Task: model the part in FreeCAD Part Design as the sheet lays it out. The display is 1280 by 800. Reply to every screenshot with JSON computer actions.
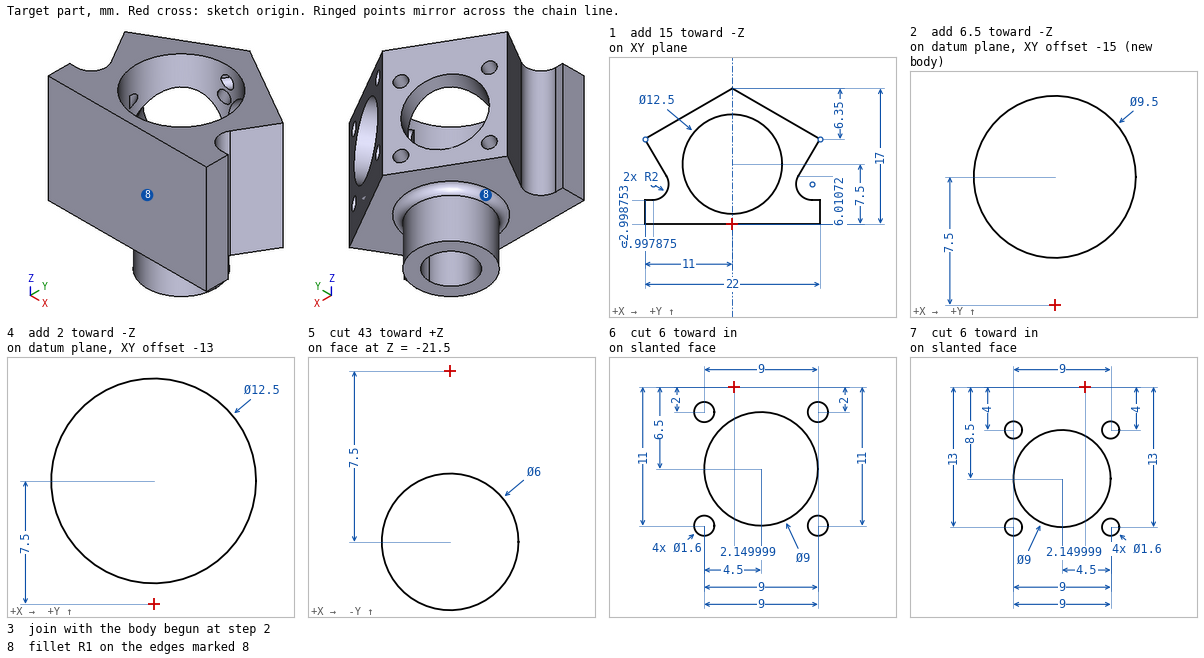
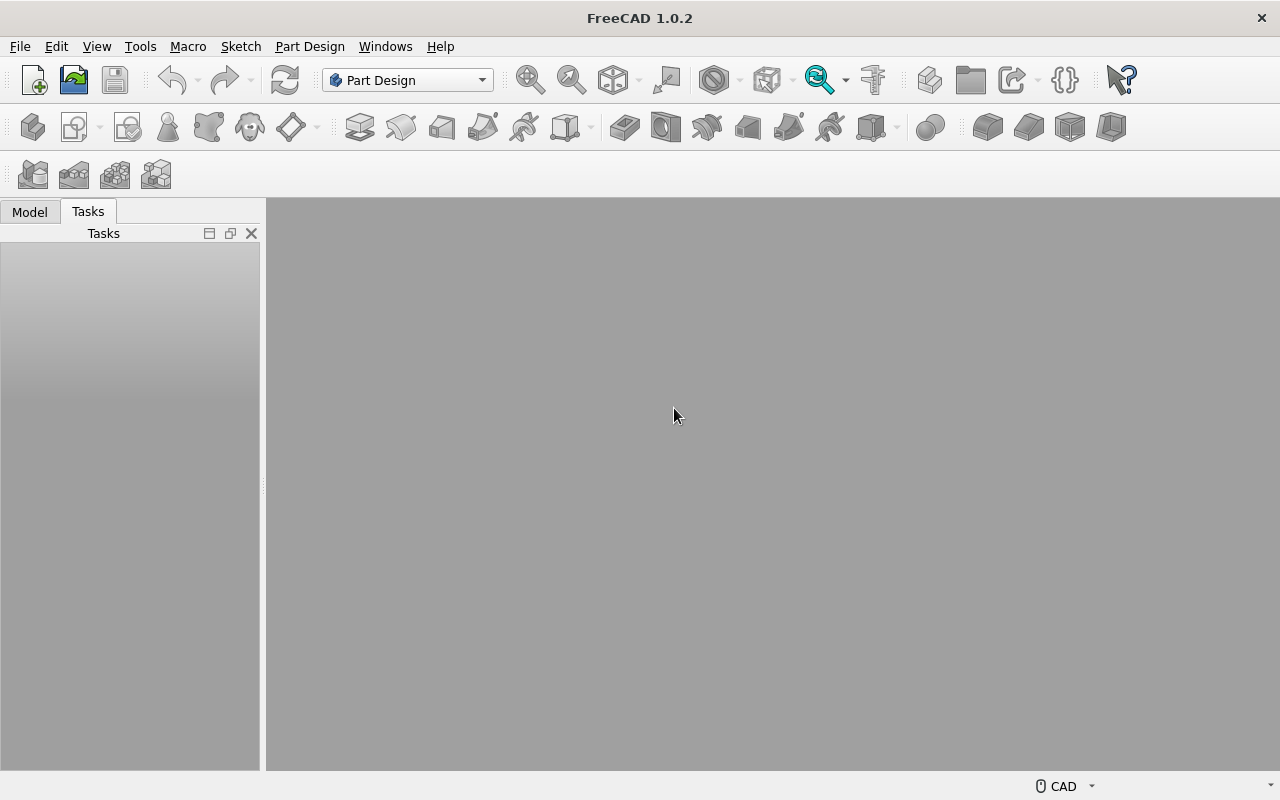
{"action": "left_click", "coordinate": [33, 80]}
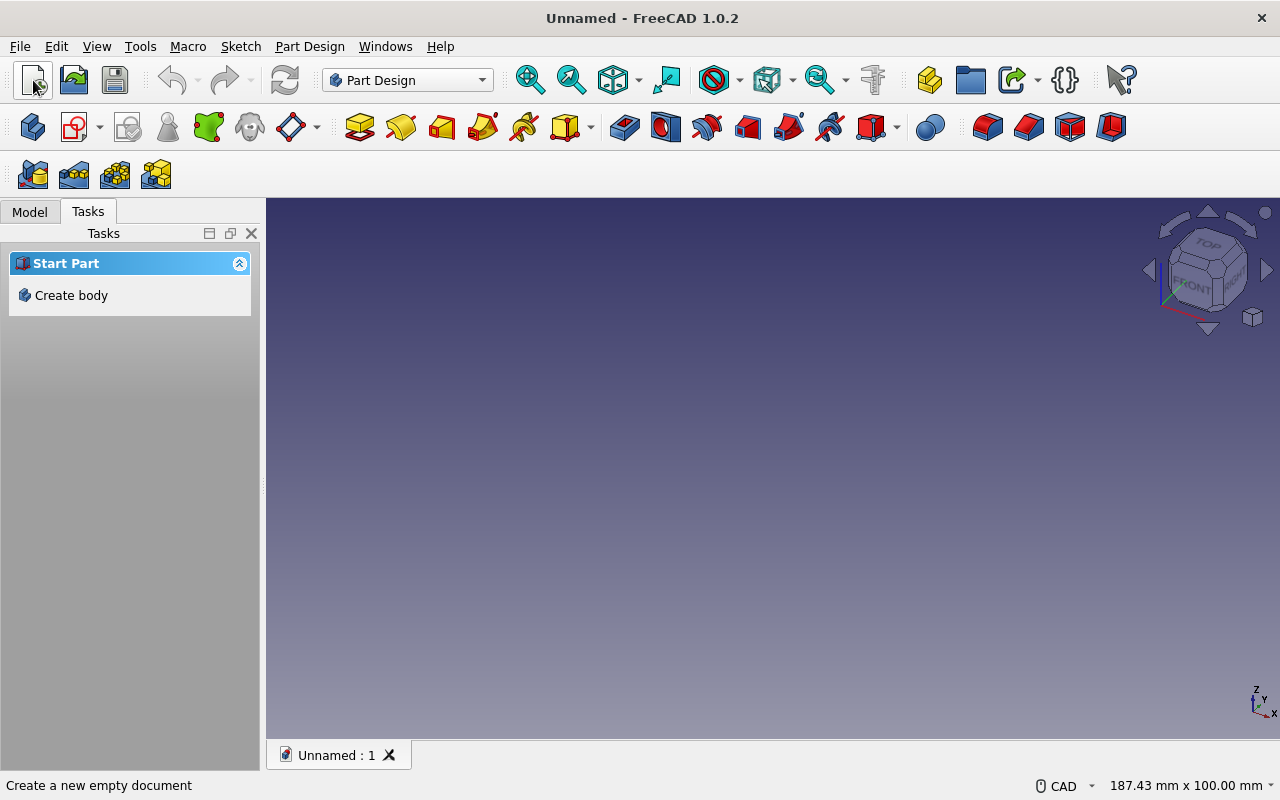
{"action": "left_click", "coordinate": [74, 128]}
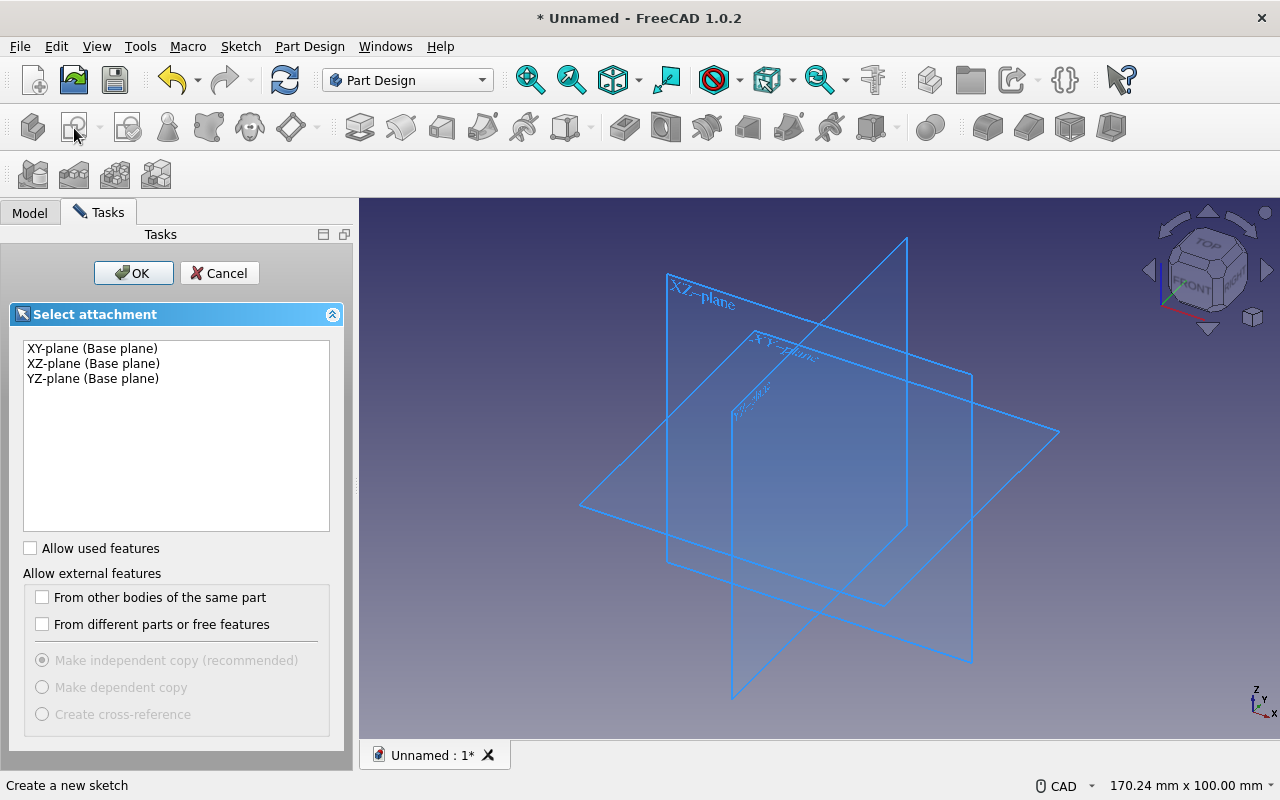
{"action": "left_click", "coordinate": [84, 348]}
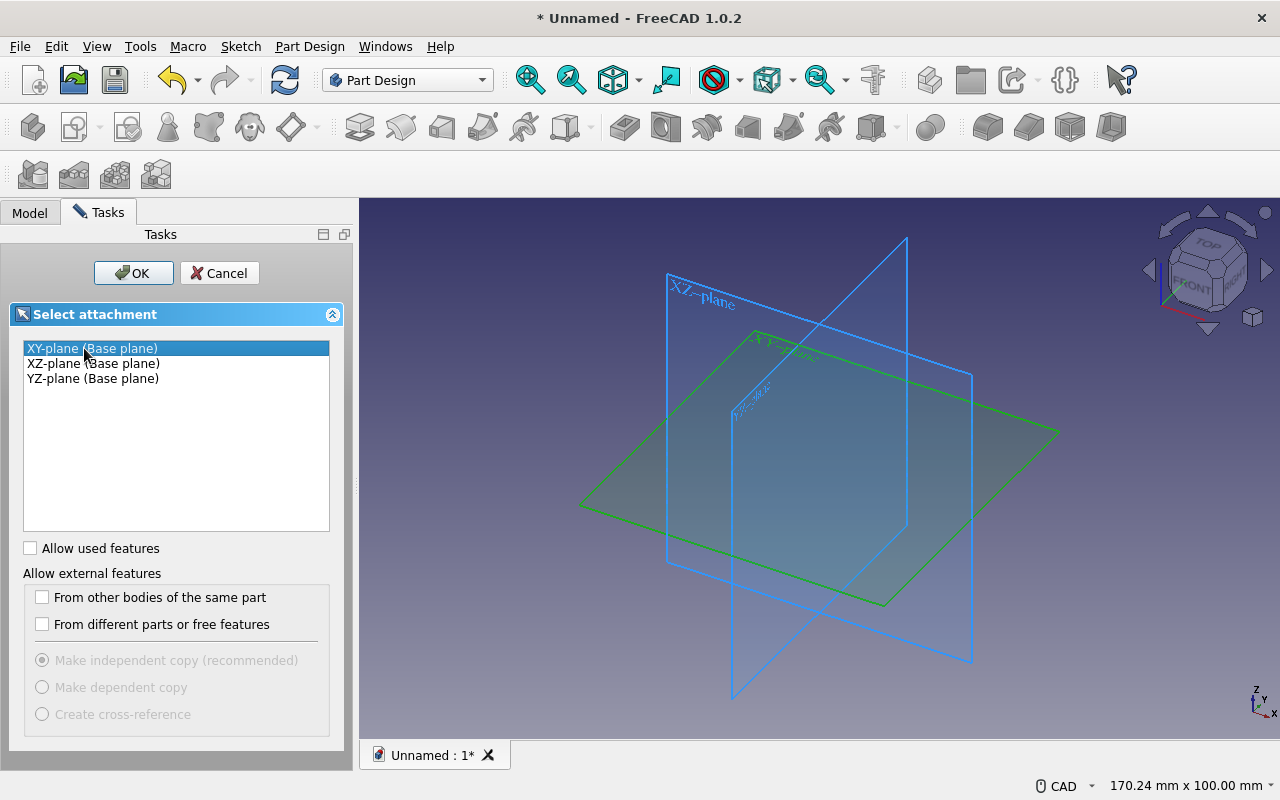
{"action": "left_click", "coordinate": [134, 273]}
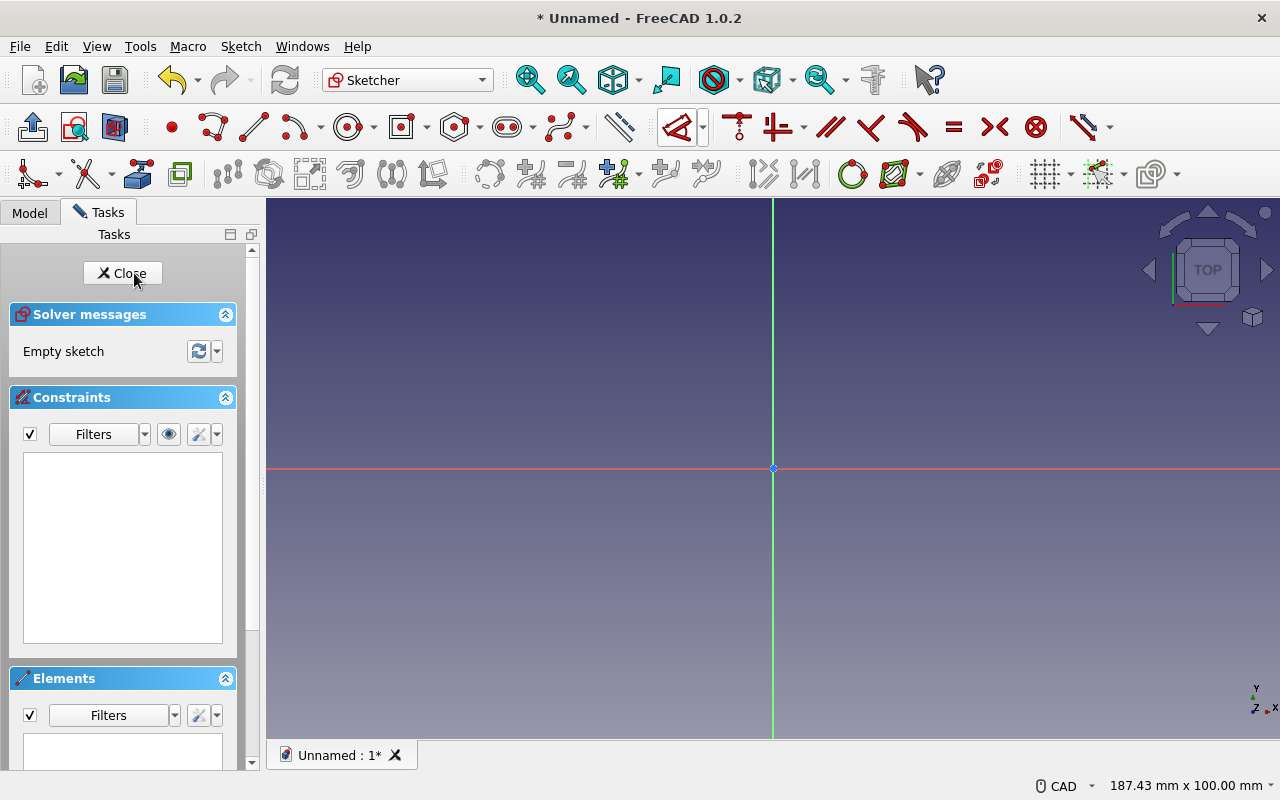
{"action": "scroll", "coordinate": [795, 407], "scroll_direction": "up", "scroll_amount": 7}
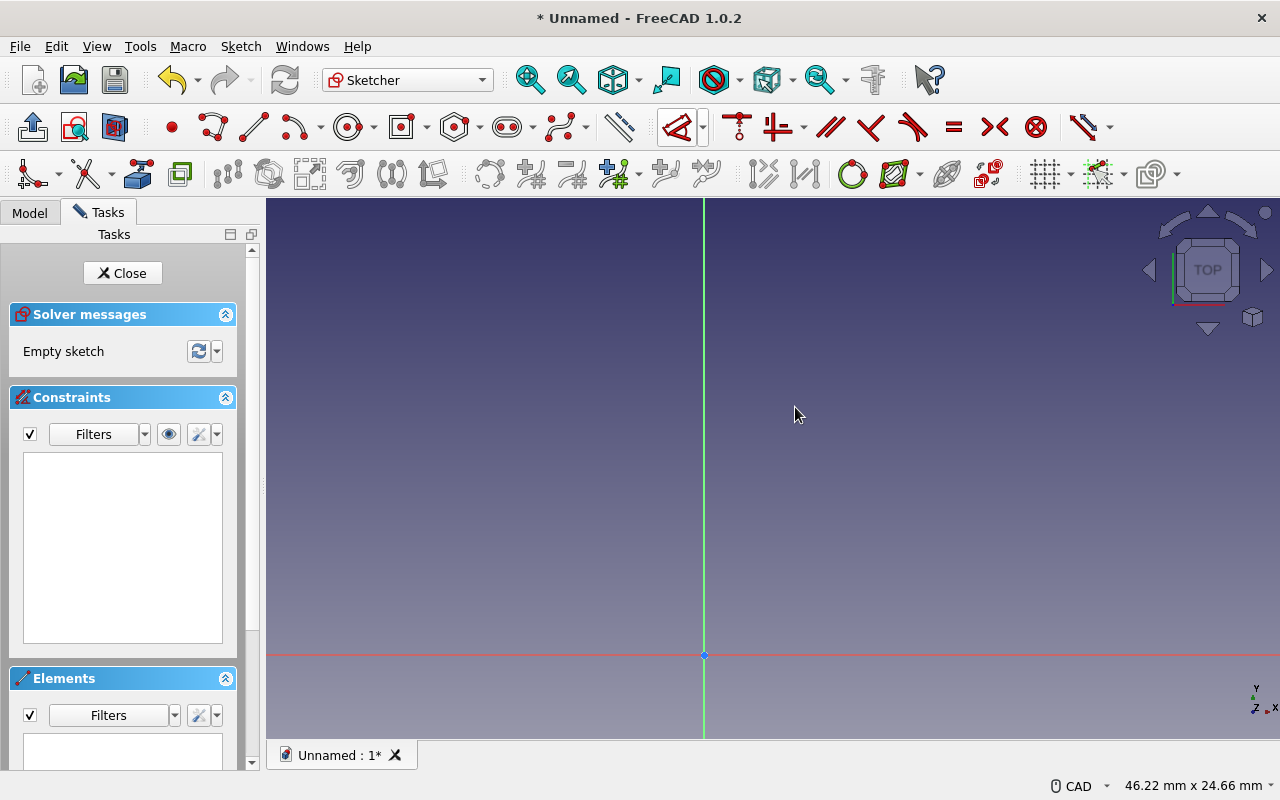
{"action": "left_click", "coordinate": [213, 128]}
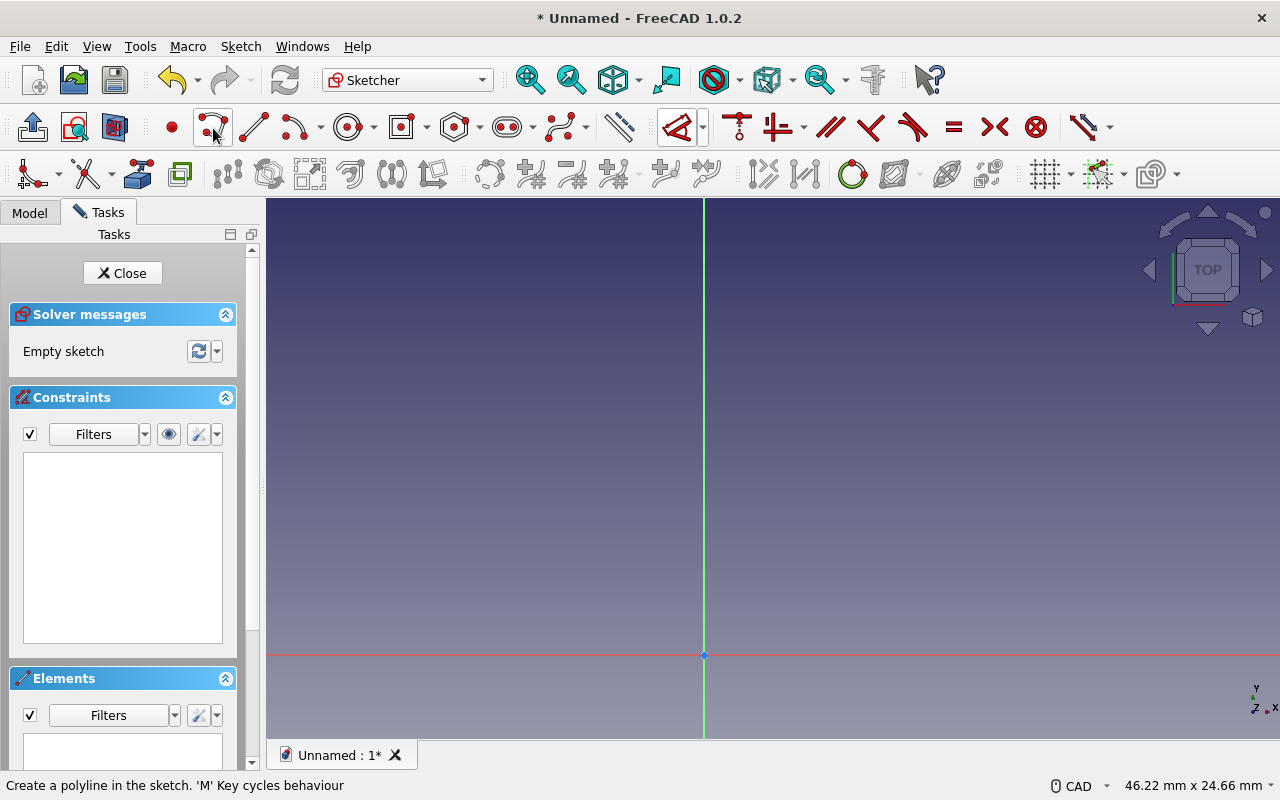
{"action": "left_click", "coordinate": [485, 589]}
{"action": "left_click", "coordinate": [463, 589]}
{"action": "left_click", "coordinate": [463, 655]}
{"action": "left_click", "coordinate": [946, 646]}
{"action": "left_click", "coordinate": [946, 589]}
{"action": "left_click", "coordinate": [924, 589]}
{"action": "right_click", "coordinate": [924, 589]}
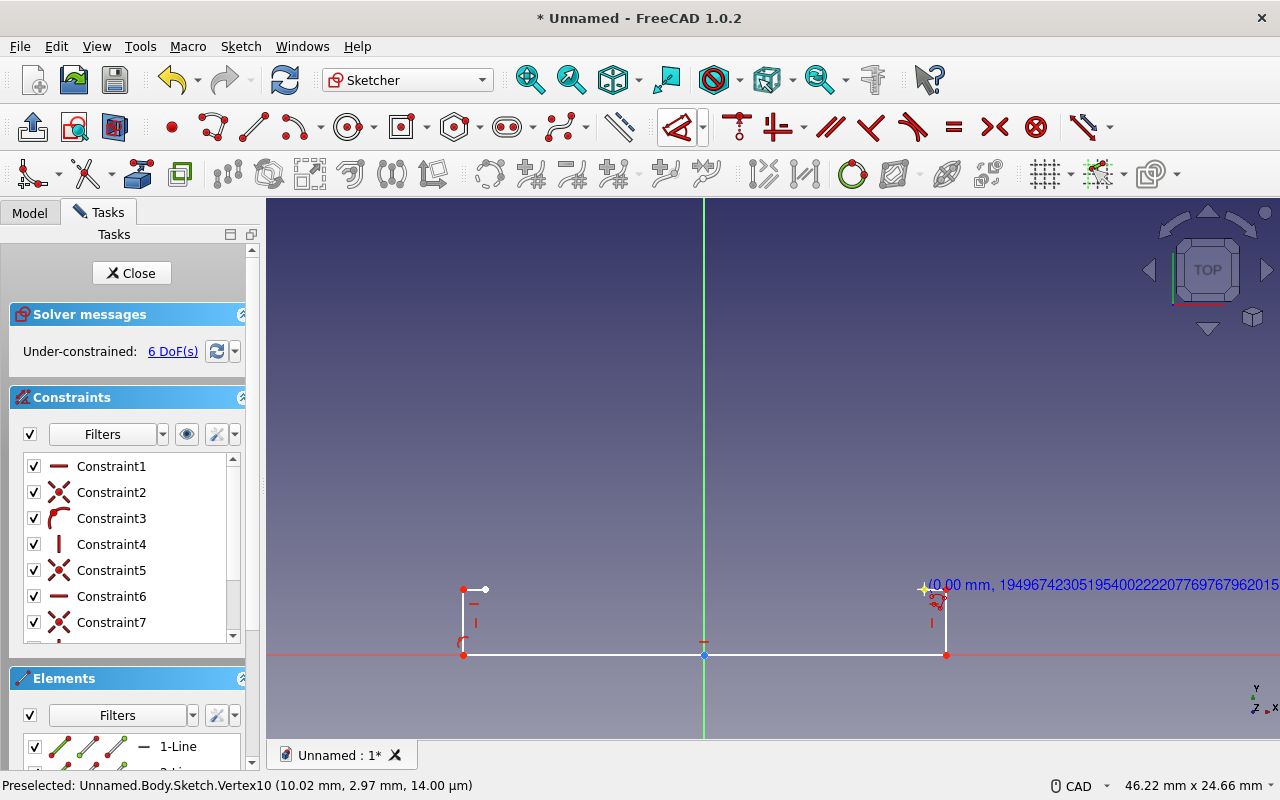
{"action": "left_click", "coordinate": [886, 523]}
{"action": "left_click", "coordinate": [945, 422]}
{"action": "left_click", "coordinate": [704, 282]}
{"action": "left_click", "coordinate": [463, 422]}
{"action": "left_click", "coordinate": [523, 523]}
{"action": "right_click", "coordinate": [523, 523]}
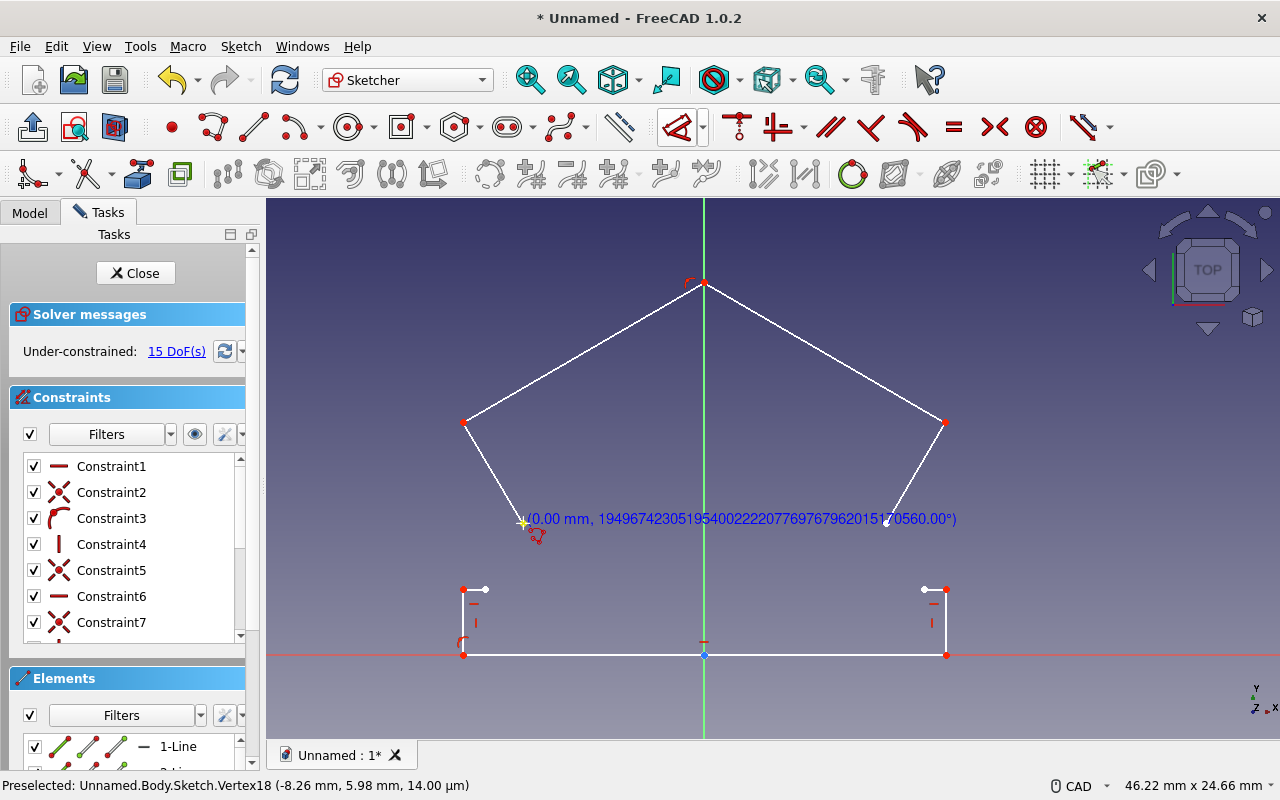
{"action": "left_click", "coordinate": [320, 128]}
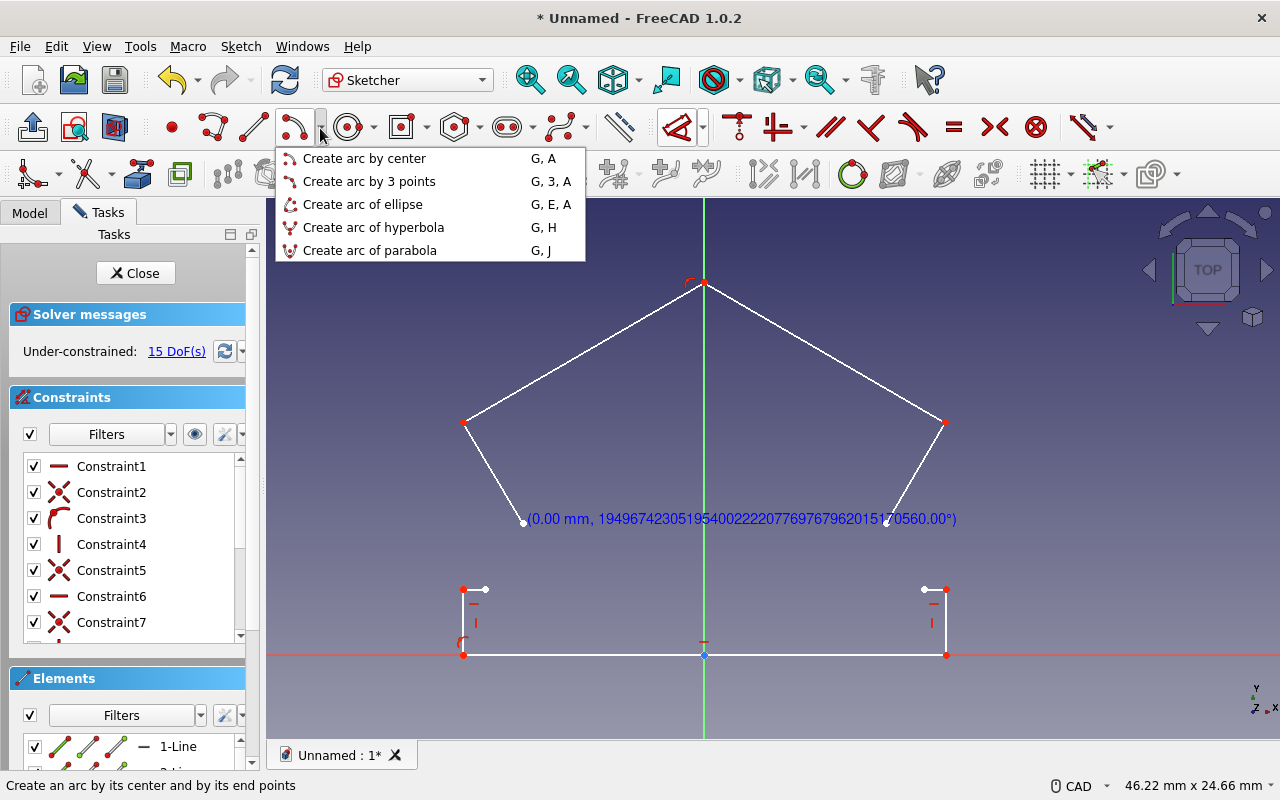
{"action": "left_click", "coordinate": [430, 182]}